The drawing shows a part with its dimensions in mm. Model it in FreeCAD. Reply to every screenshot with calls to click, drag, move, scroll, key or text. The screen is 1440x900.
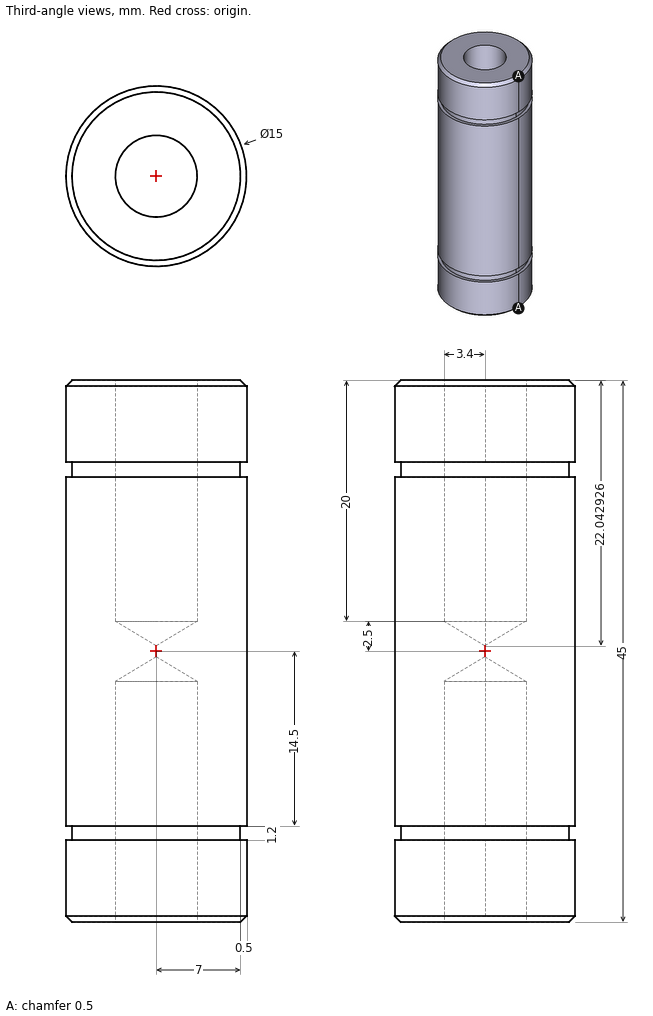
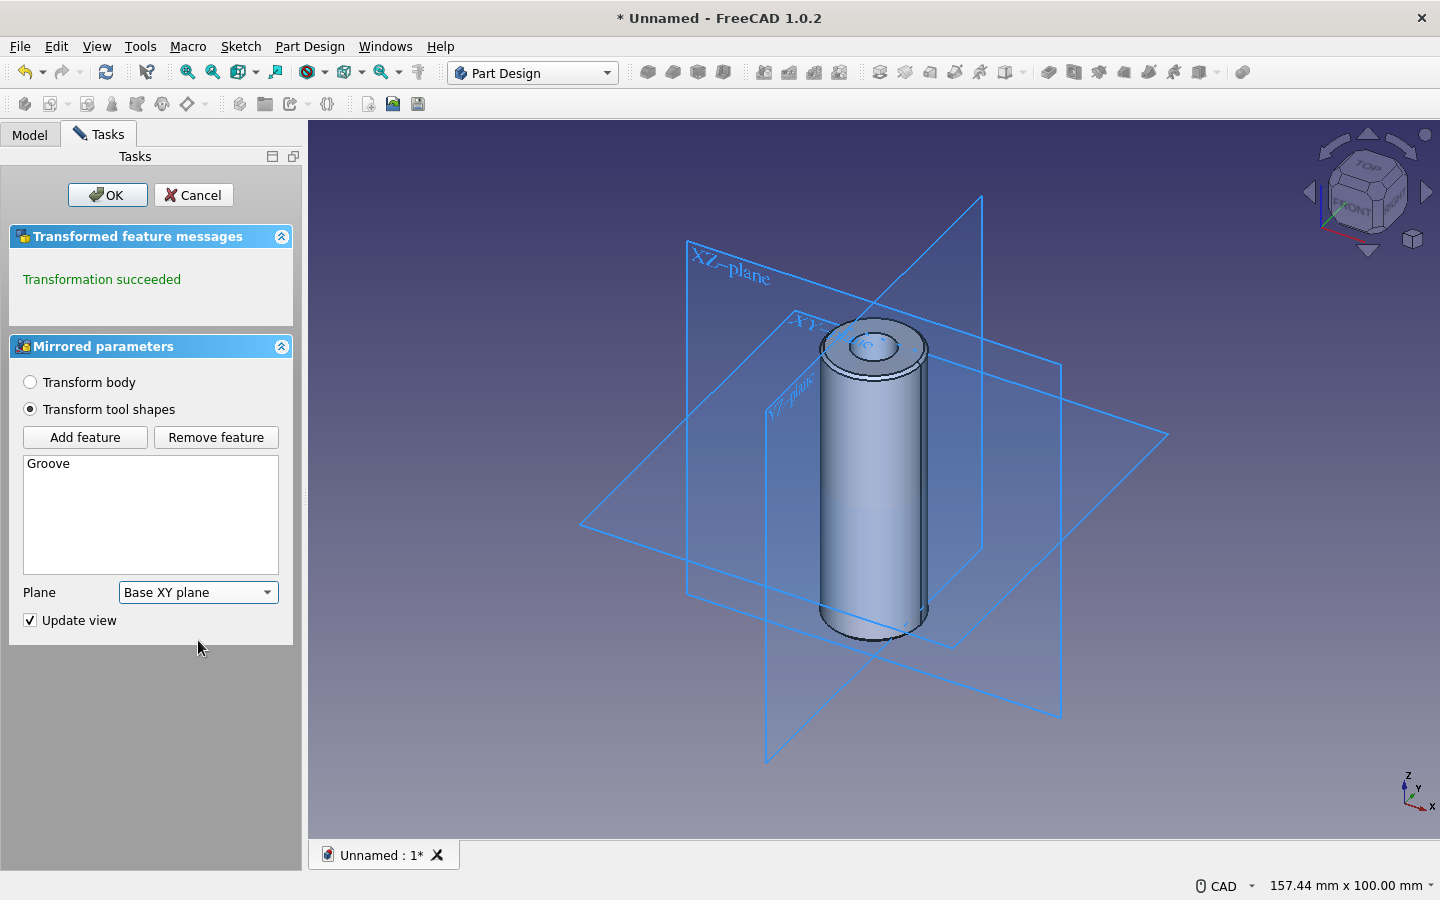
click(108, 195)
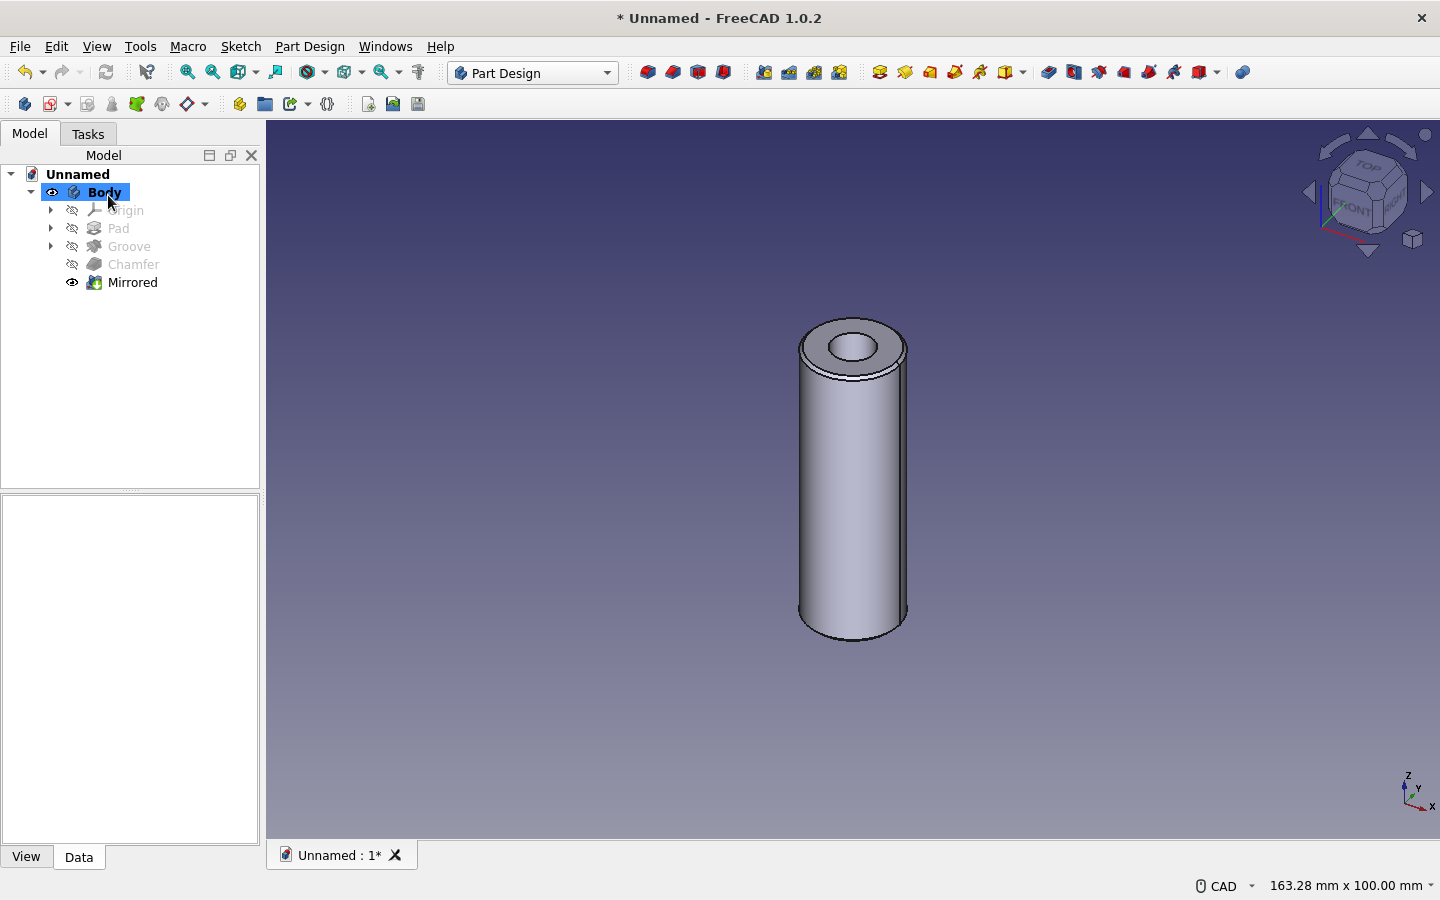
click(50, 104)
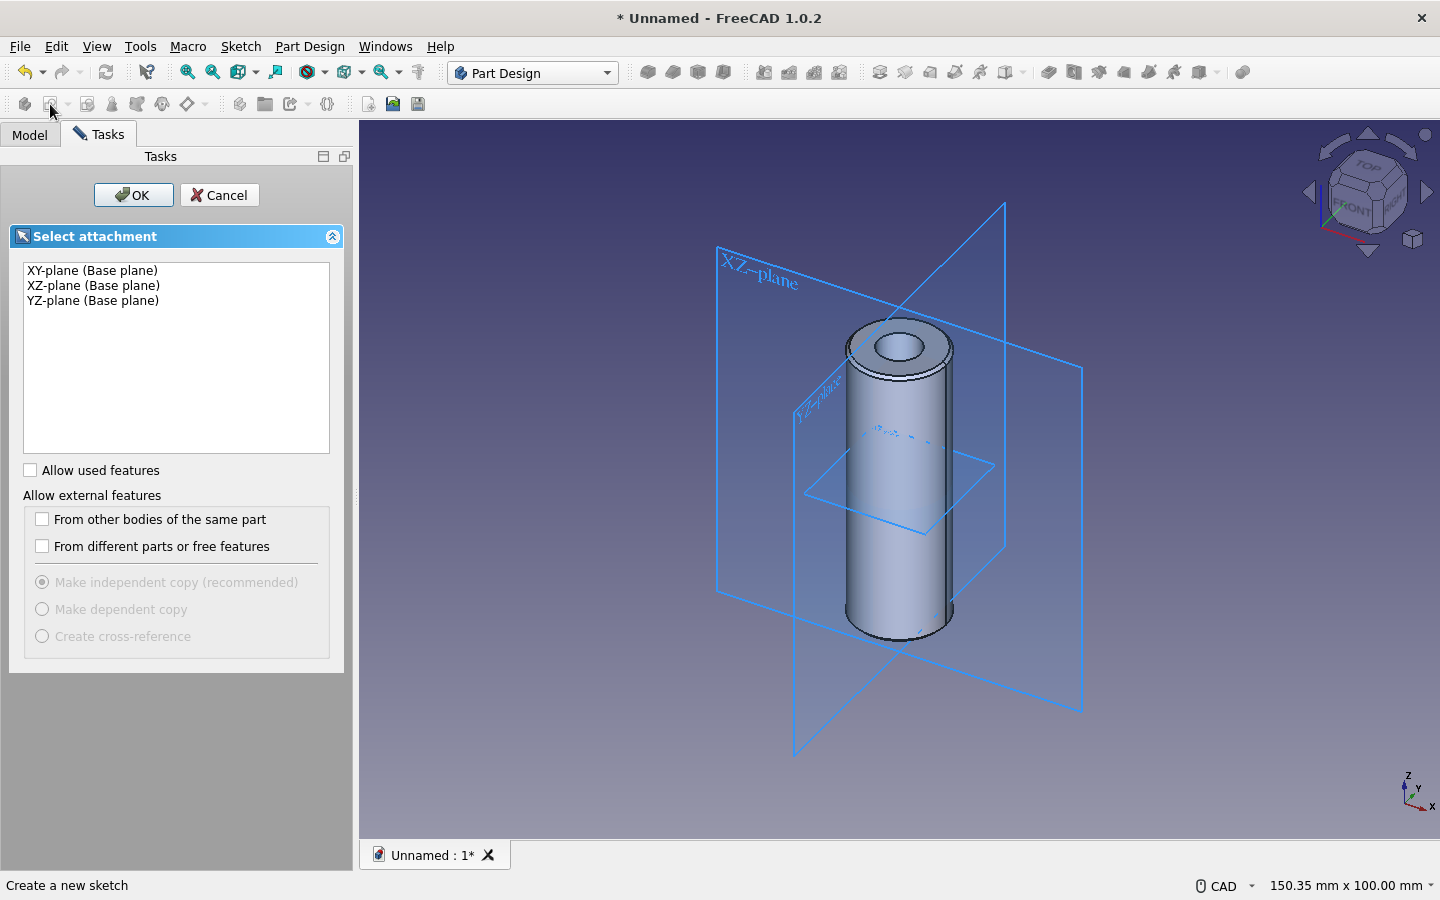
click(84, 286)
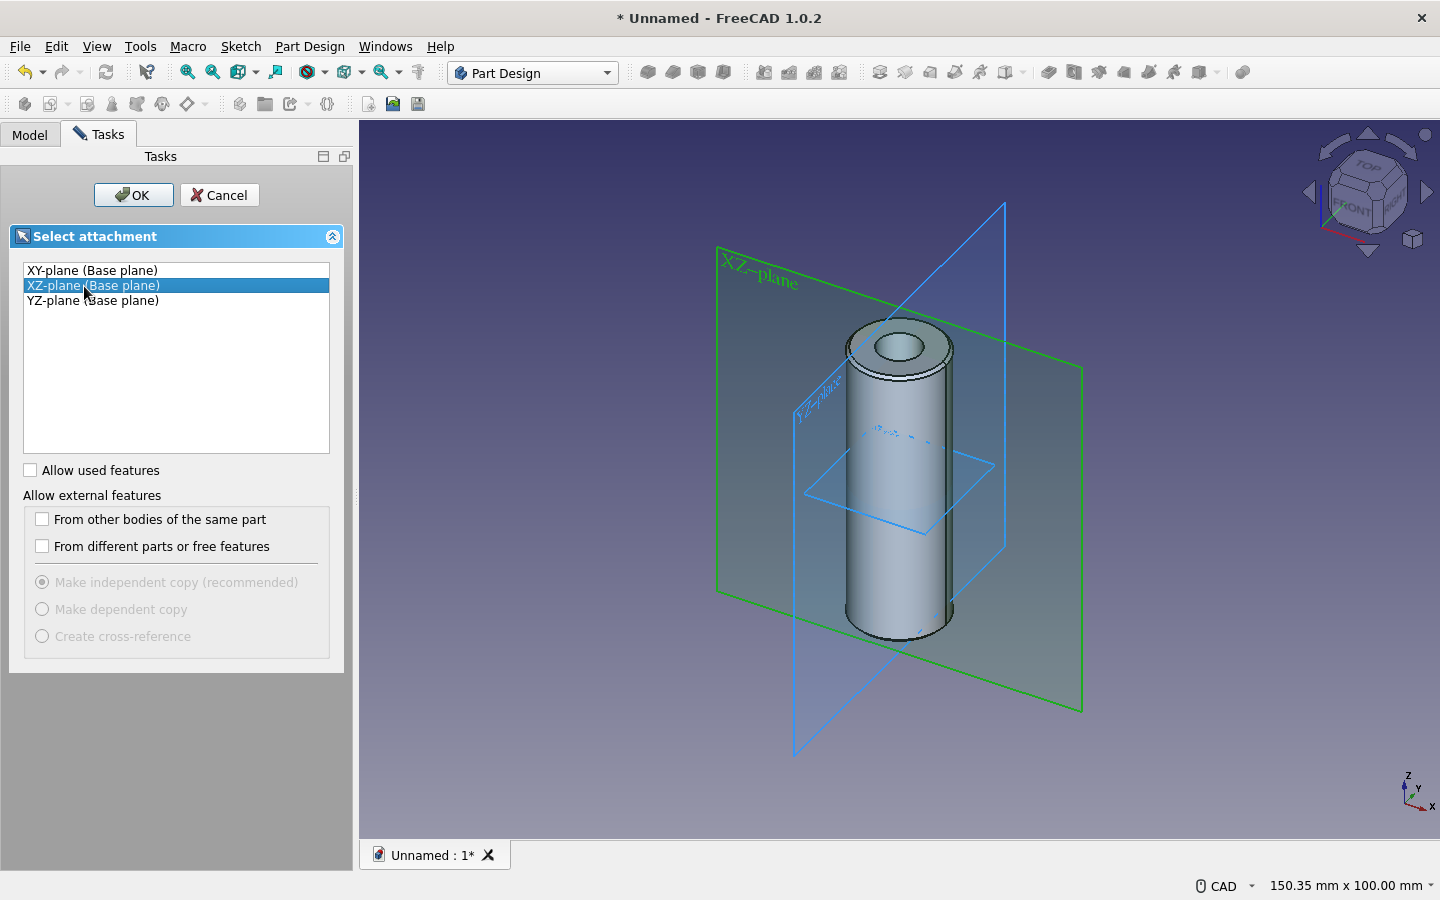
click(134, 195)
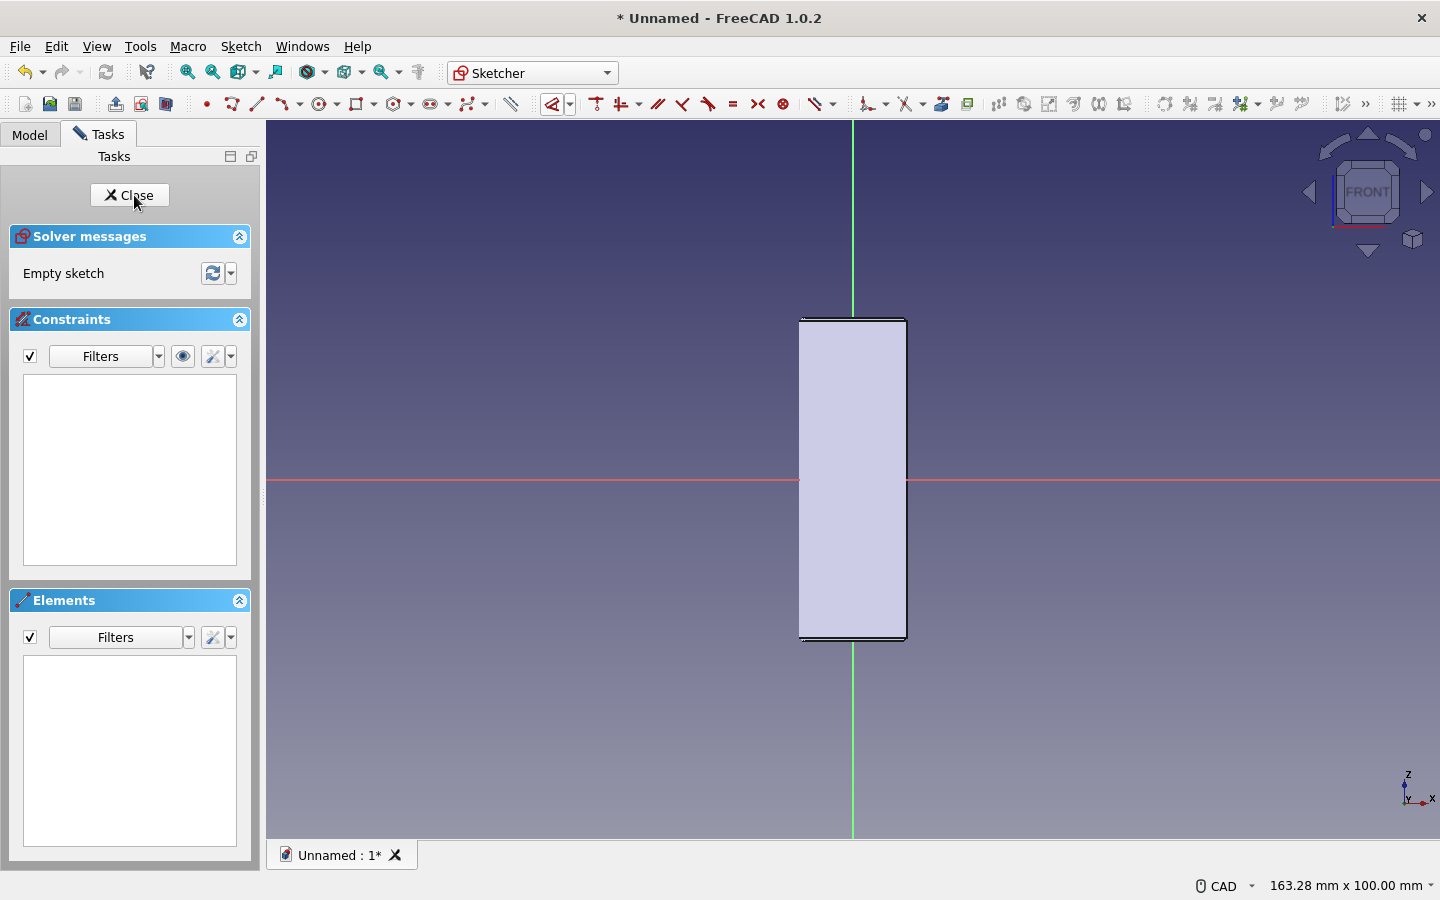
click(166, 104)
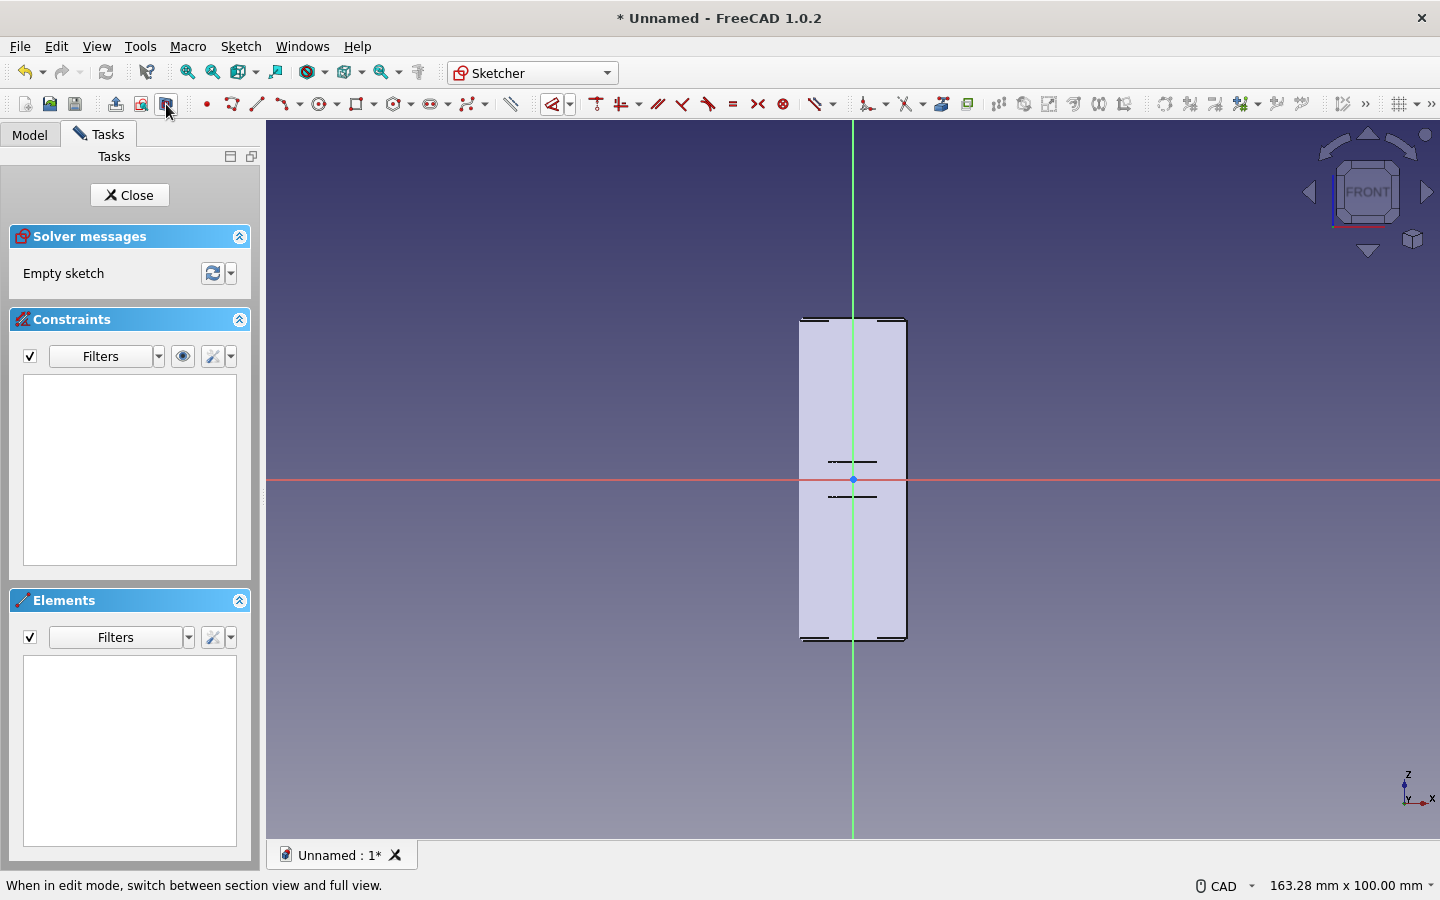
scroll(911, 594, up, 15)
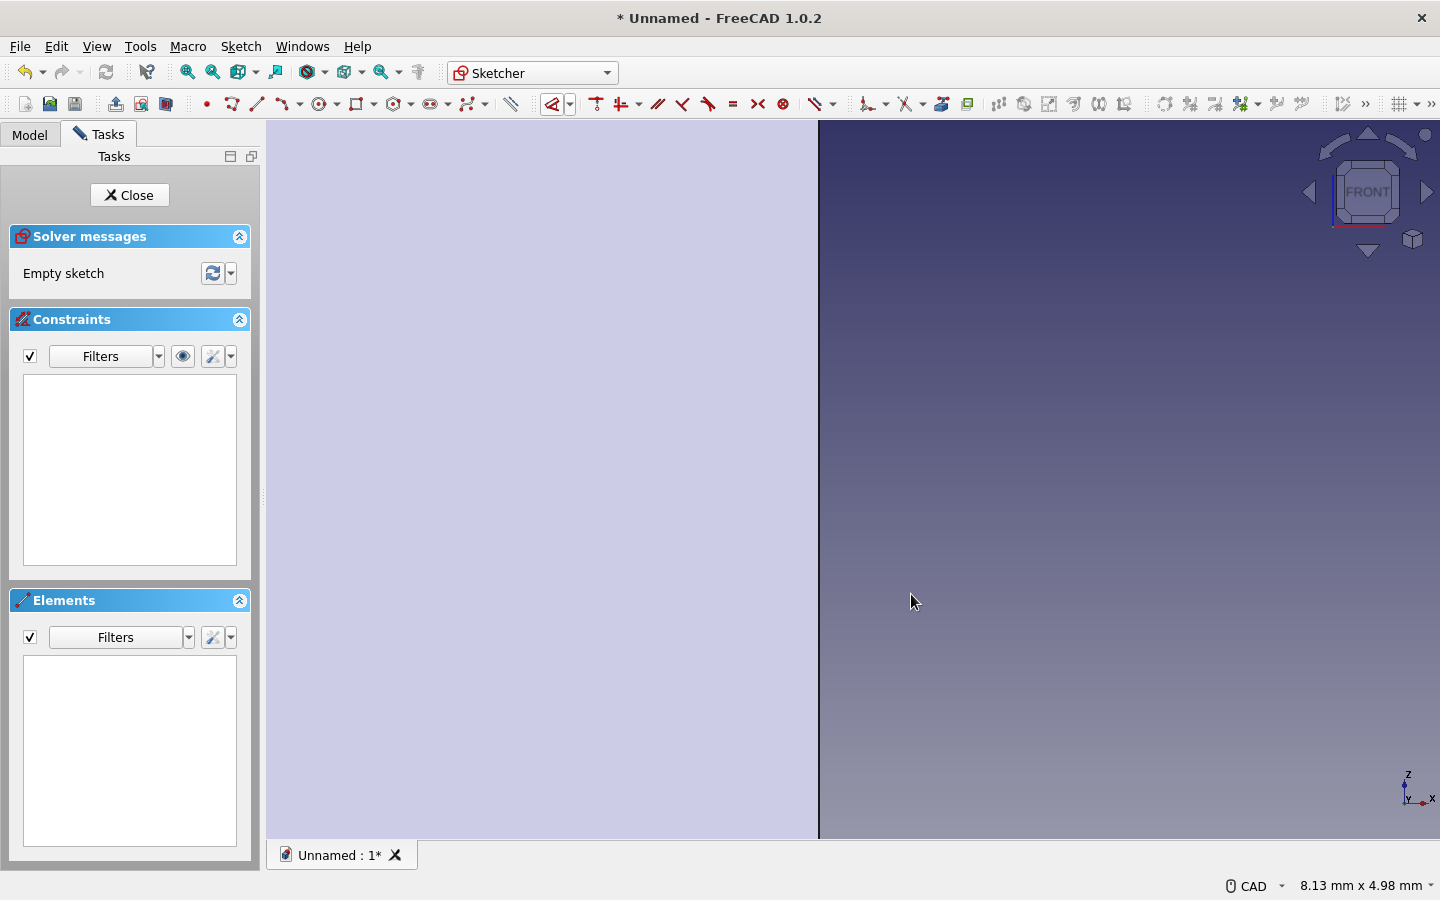
scroll(781, 452, up, 5)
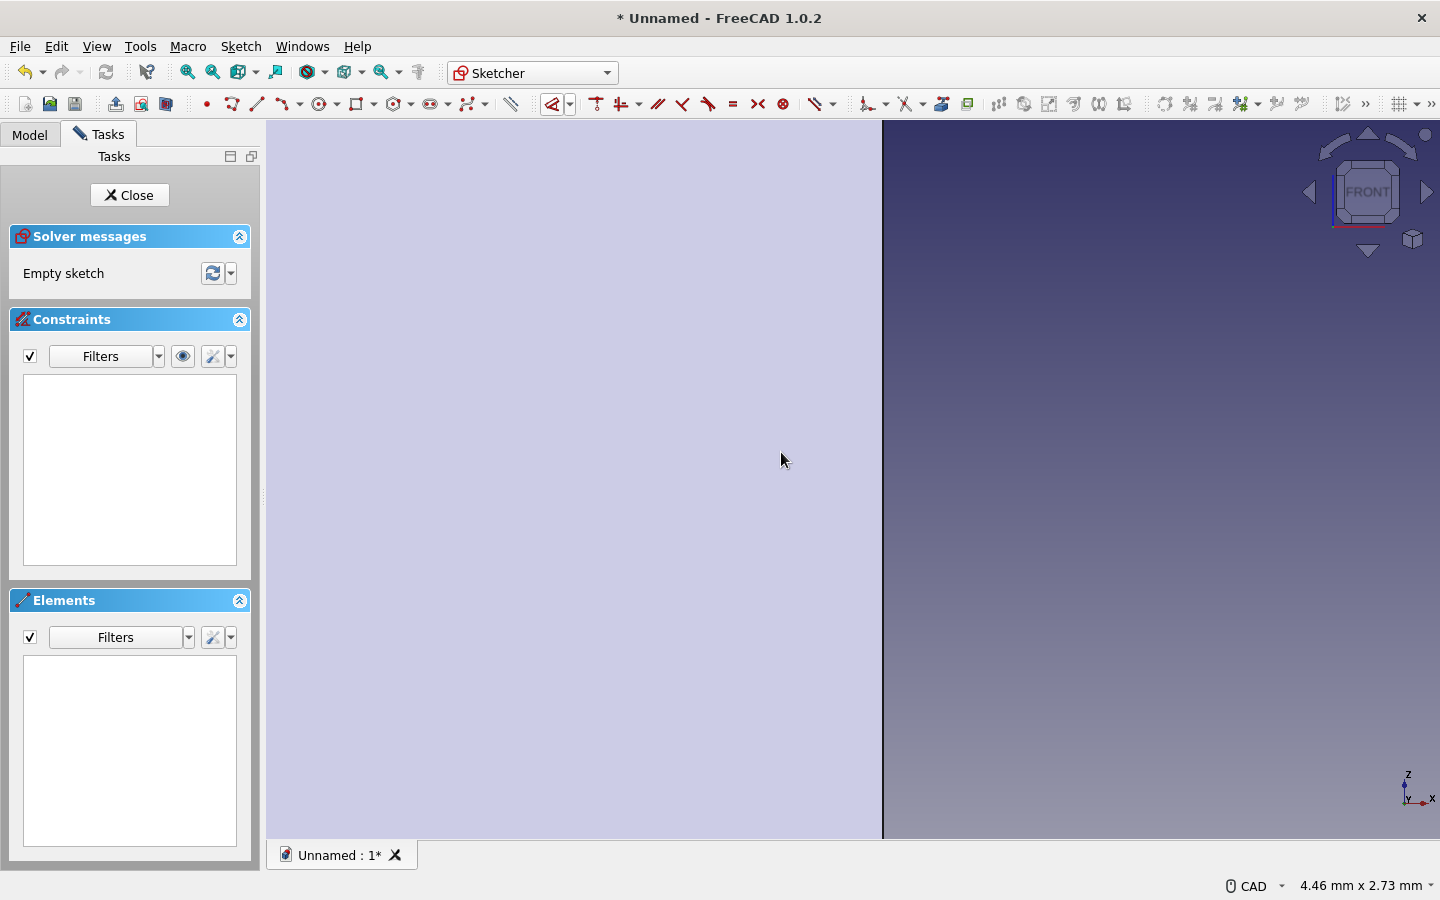
key(g)
key(r)